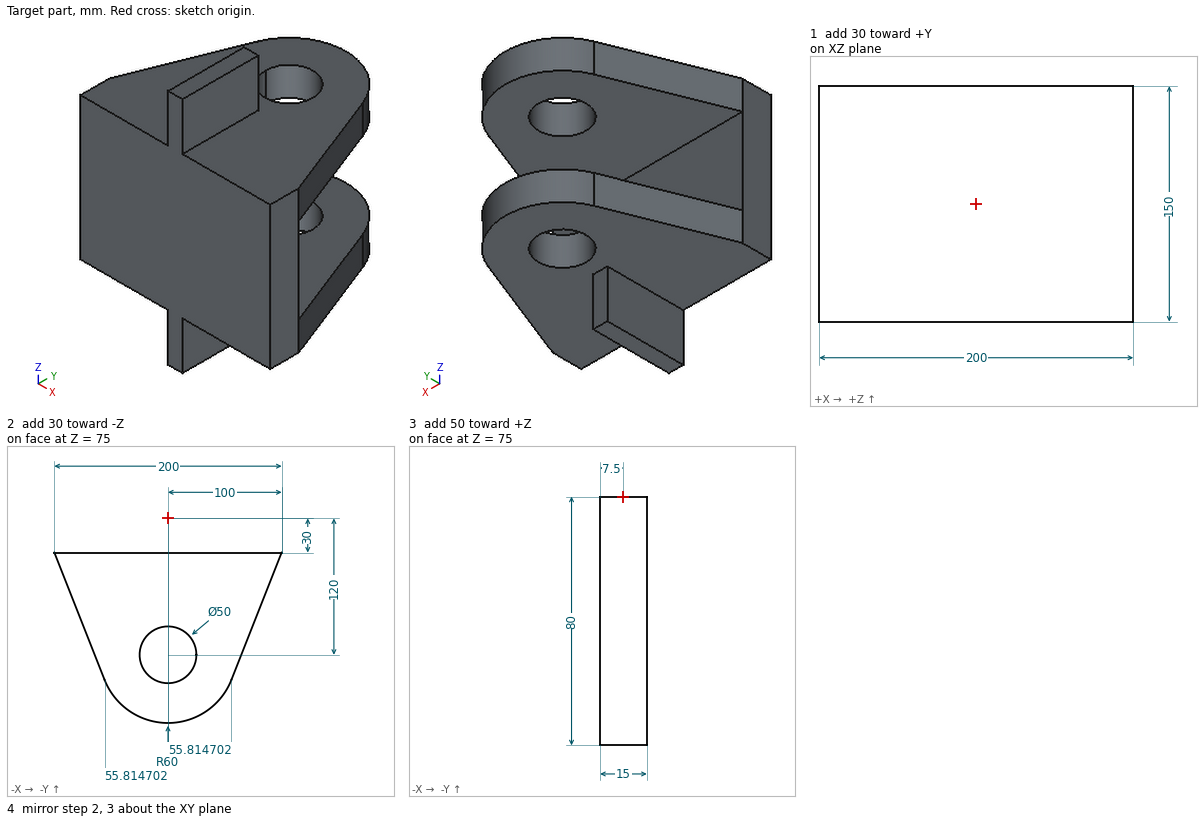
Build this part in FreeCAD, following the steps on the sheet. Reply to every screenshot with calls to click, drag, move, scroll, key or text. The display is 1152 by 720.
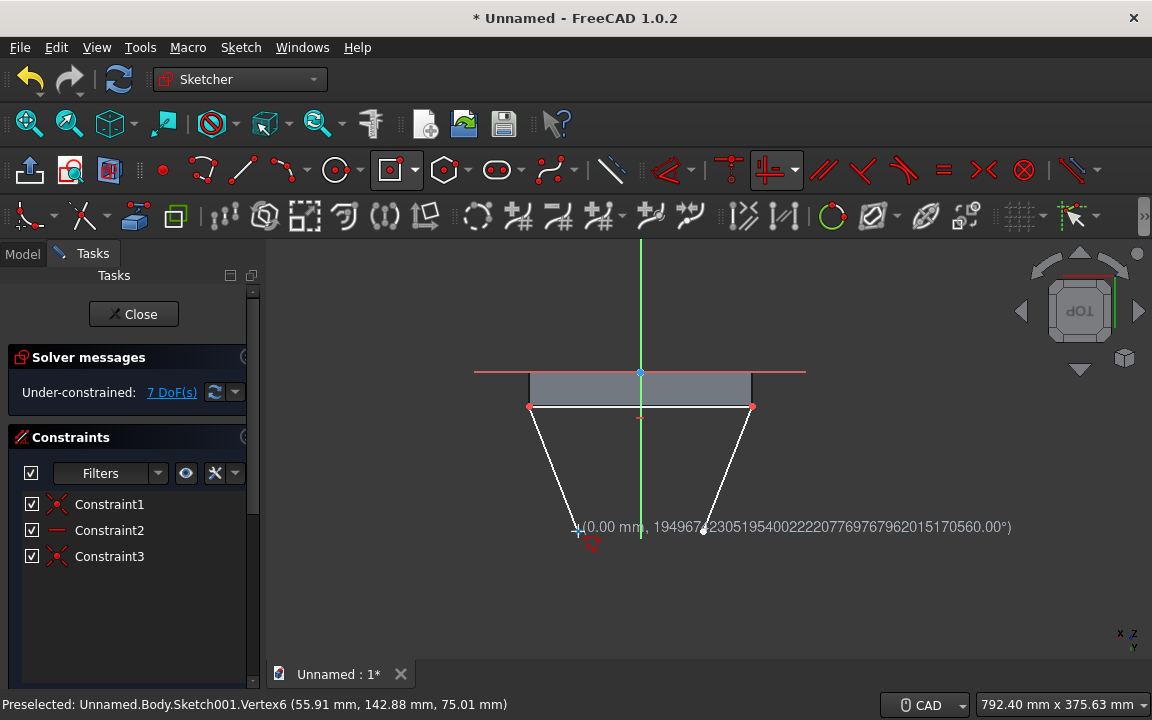
click(284, 170)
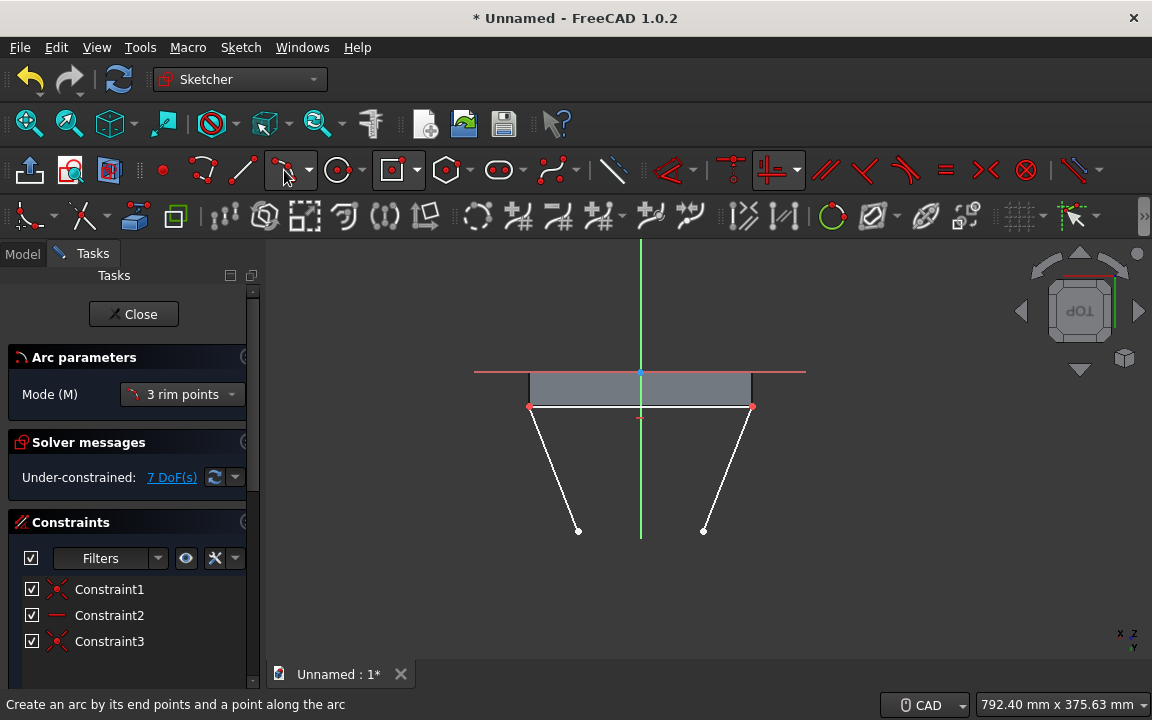
click(578, 532)
click(703, 532)
click(625, 572)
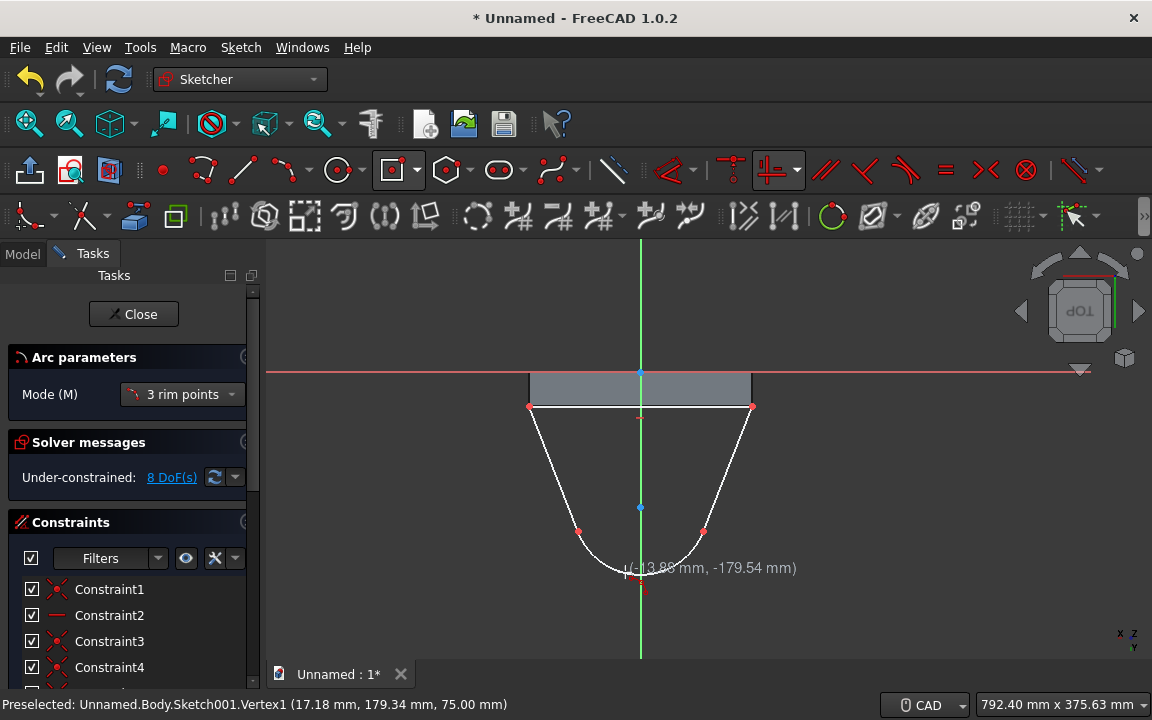
key(g)
key(c)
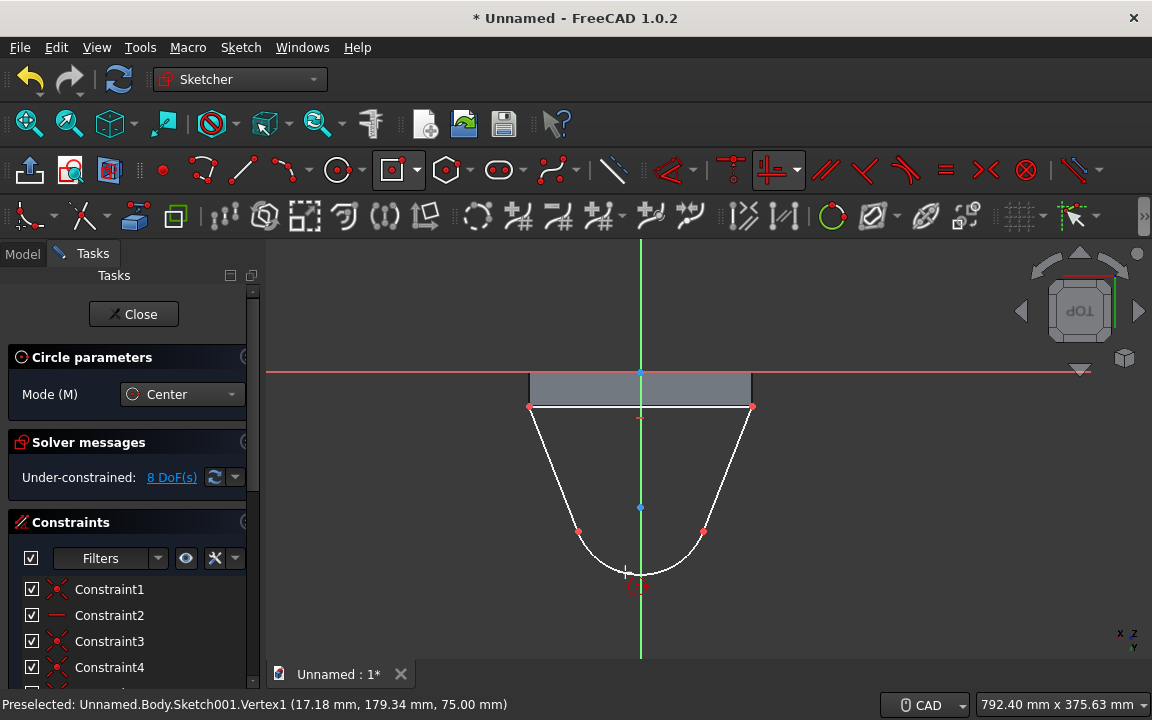
click(641, 506)
click(660, 487)
key(Escape)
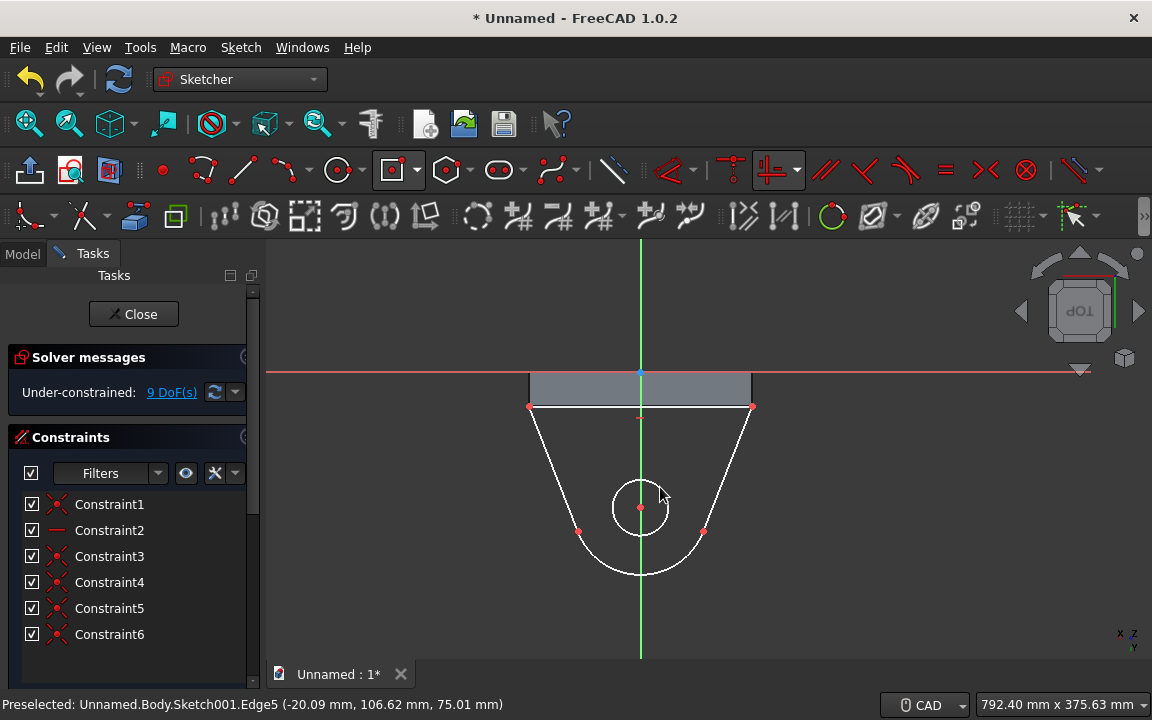
click(641, 508)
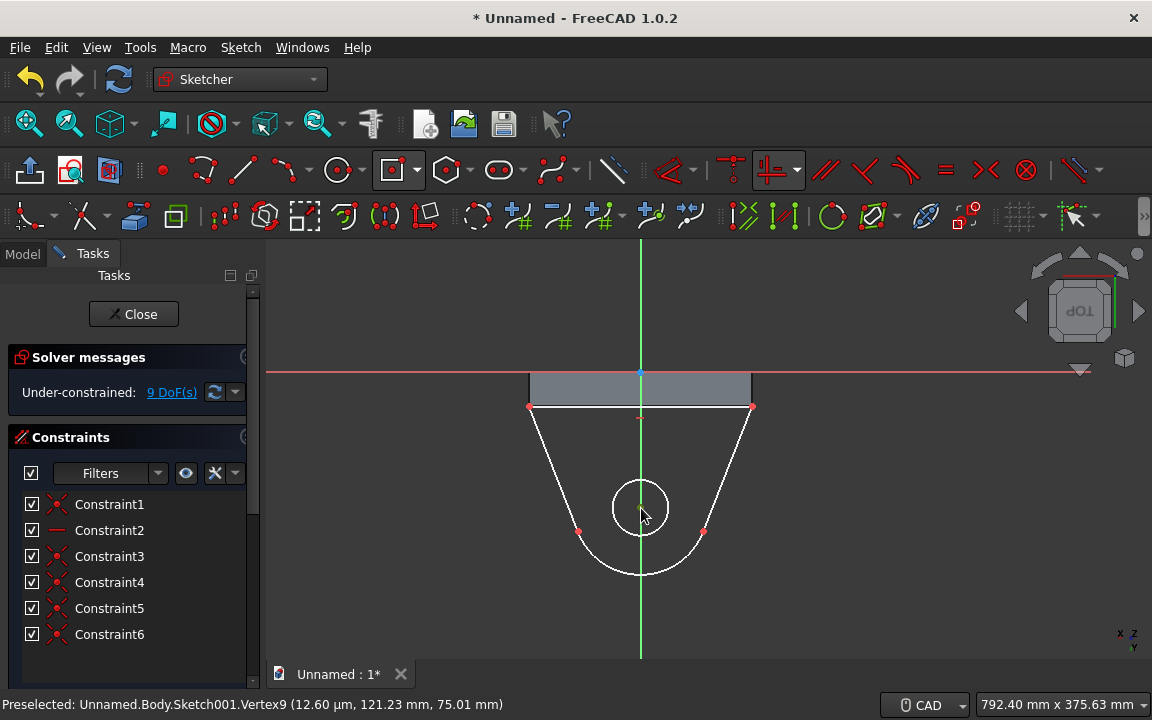
click(641, 605)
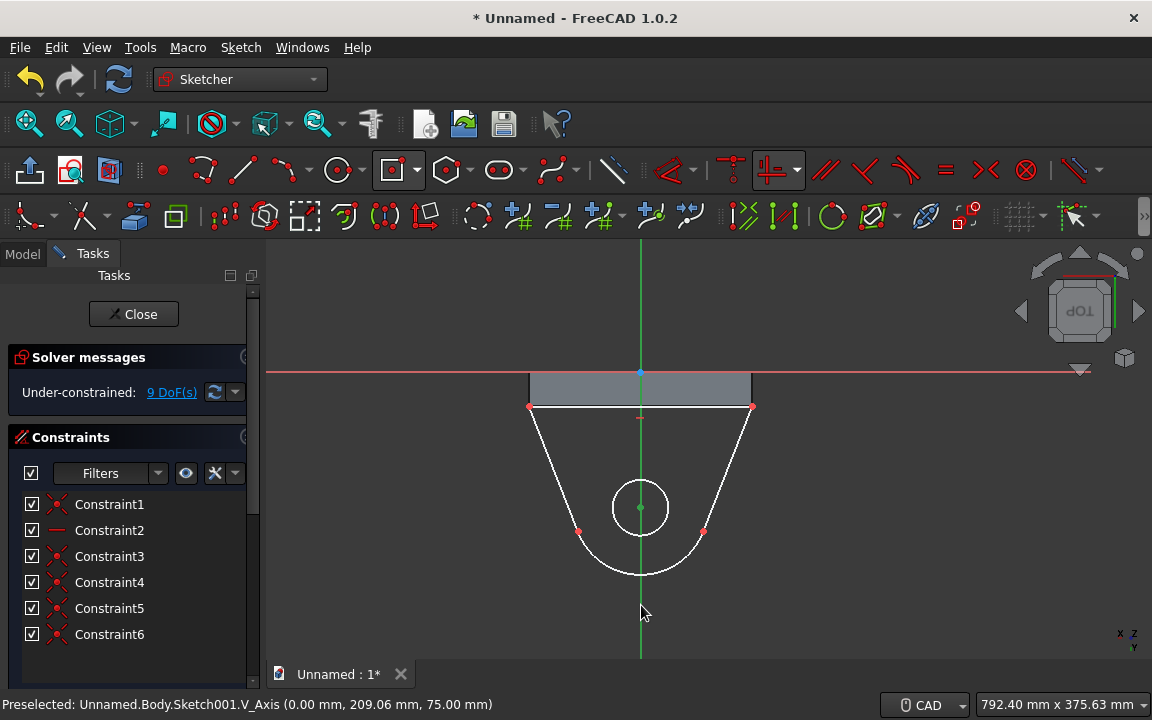
key(c)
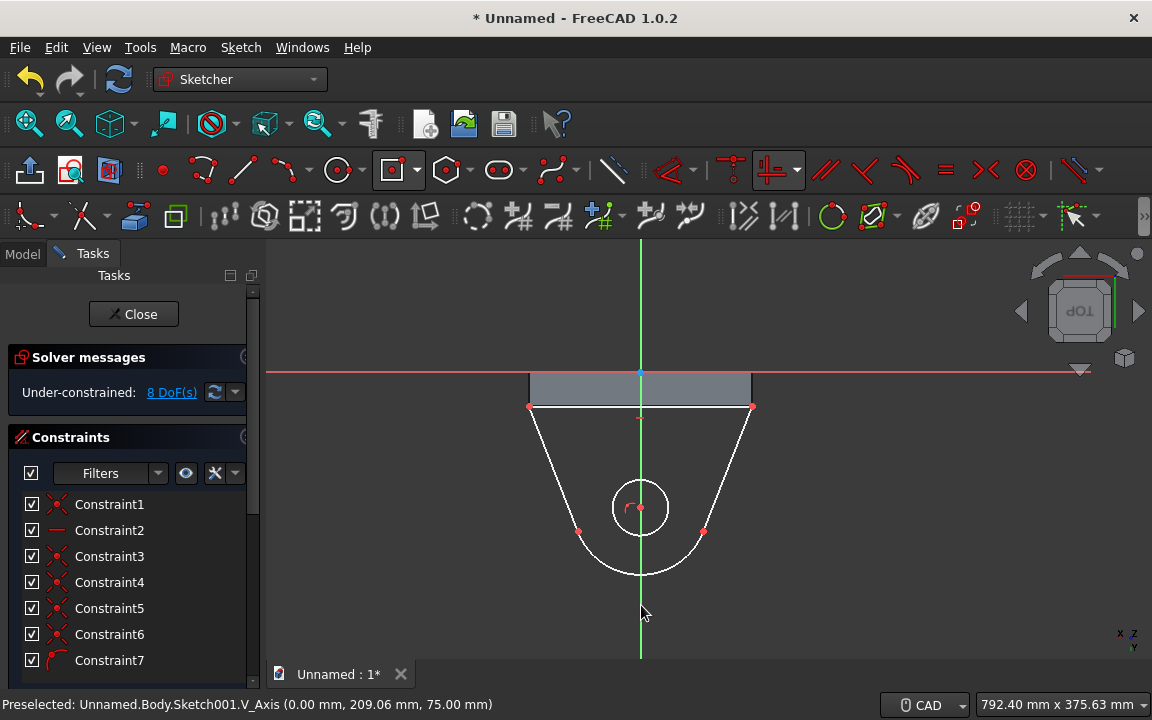
key(d)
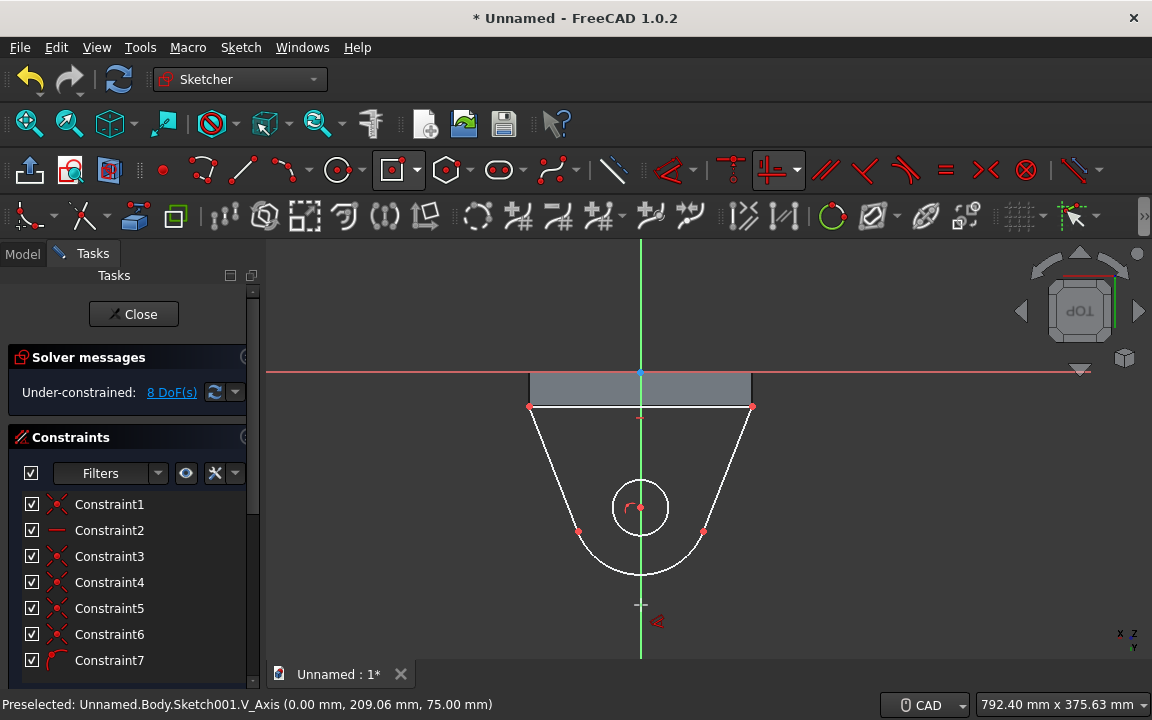
click(610, 567)
click(595, 595)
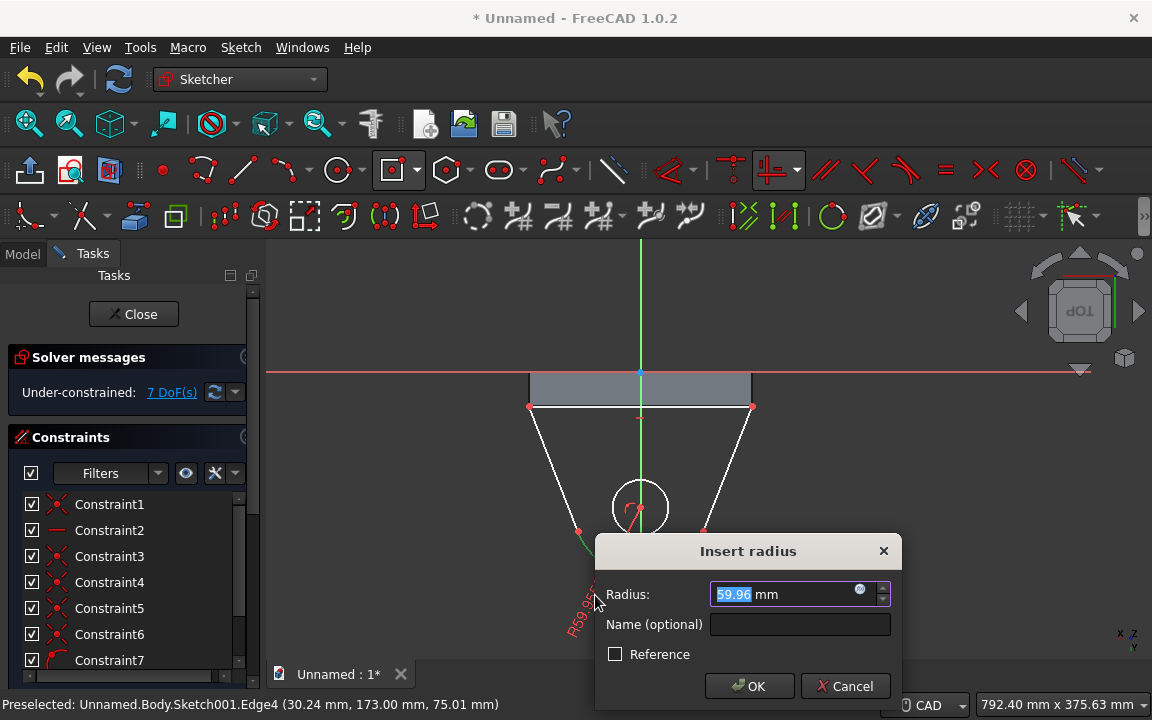
text(60)
key(Return)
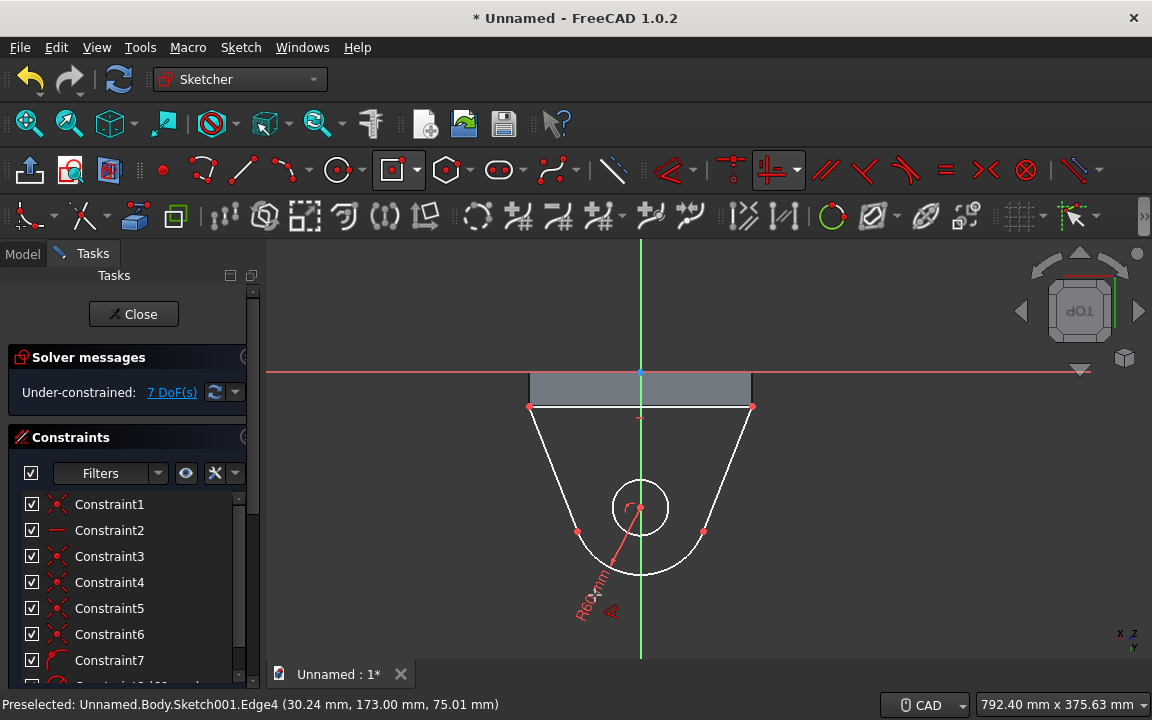
click(660, 488)
click(682, 465)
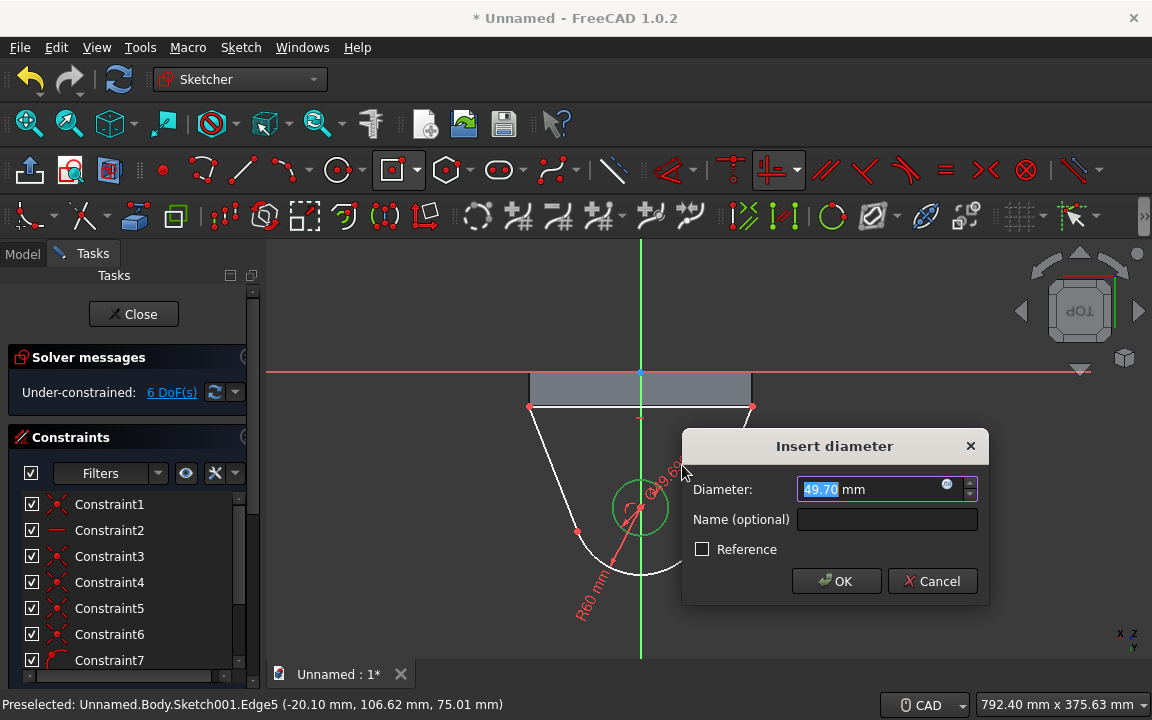
text(50)
key(Return)